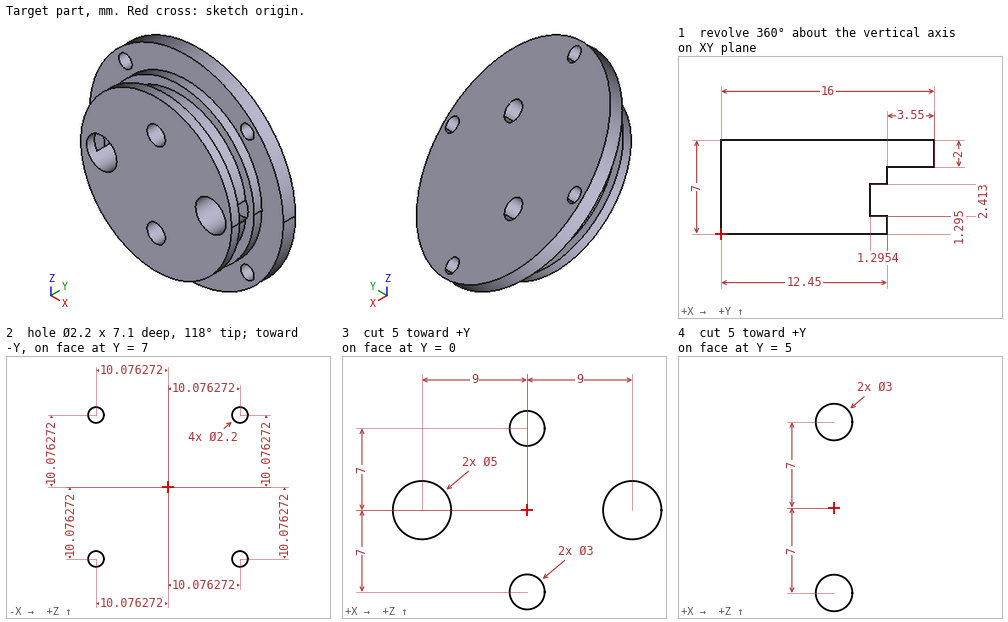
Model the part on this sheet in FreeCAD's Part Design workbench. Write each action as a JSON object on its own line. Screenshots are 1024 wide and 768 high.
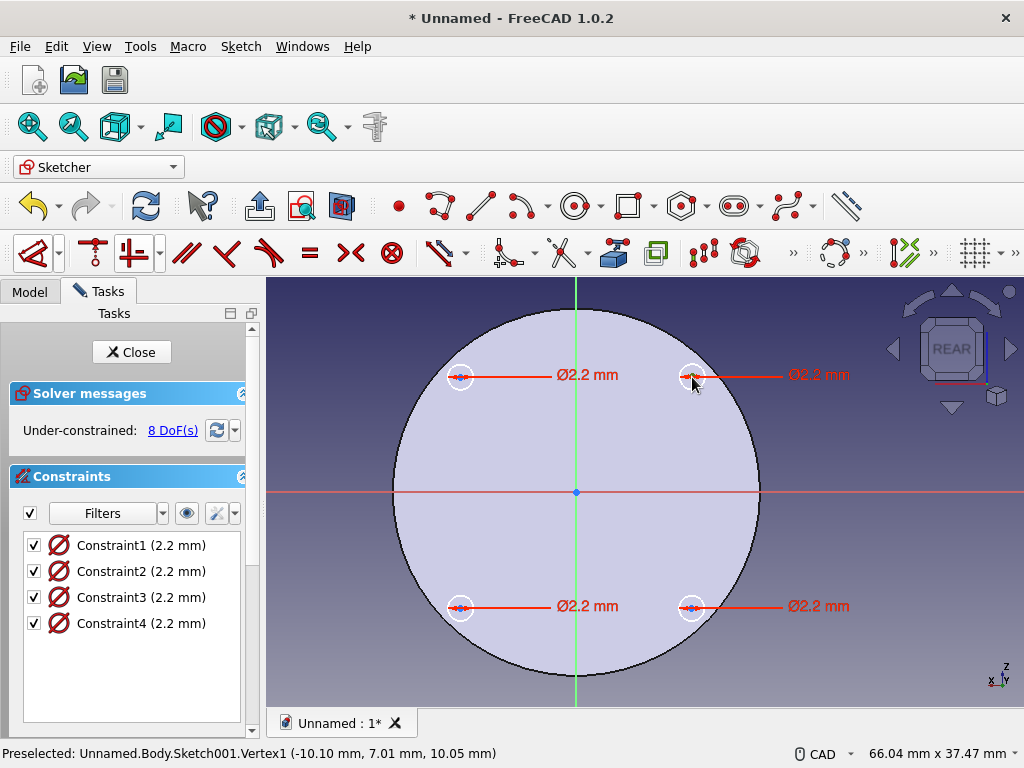
{"action": "key", "text": "l"}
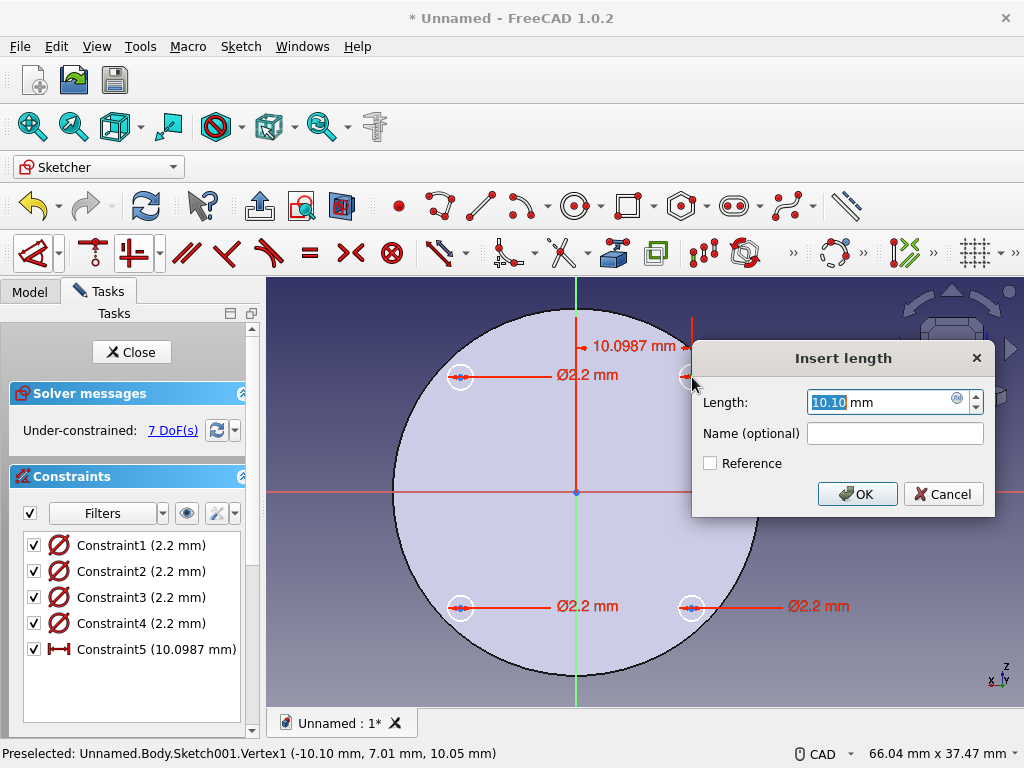
{"action": "type", "text": "10.076272"}
{"action": "key", "text": "Return"}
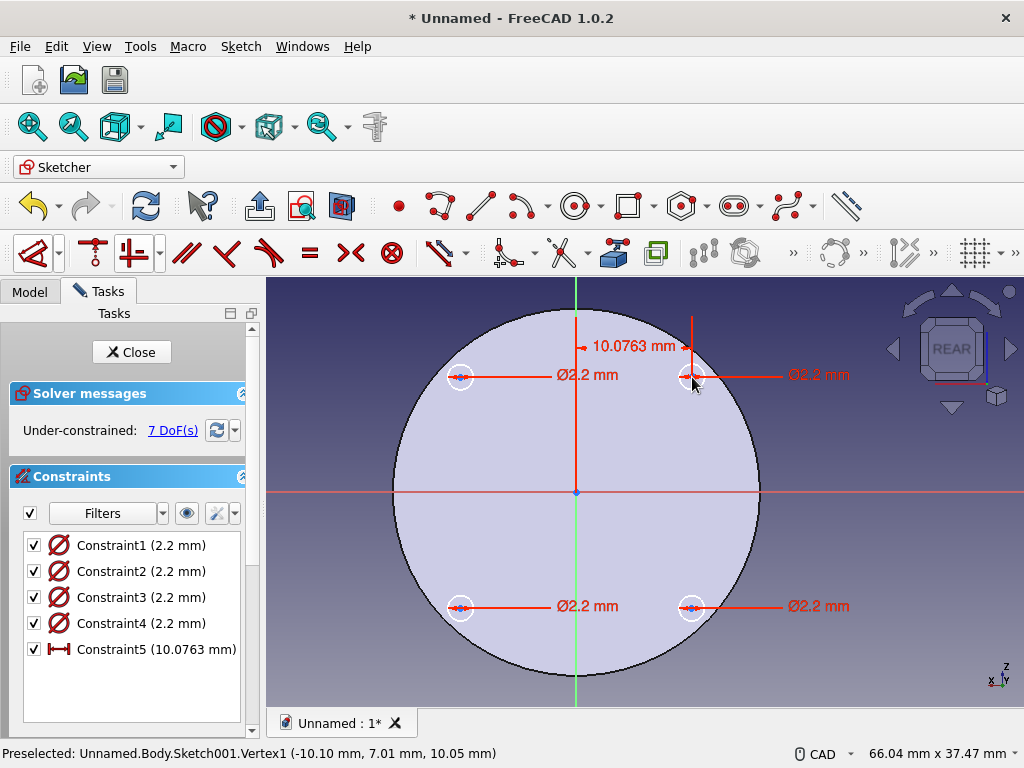
{"action": "left_click", "coordinate": [692, 377]}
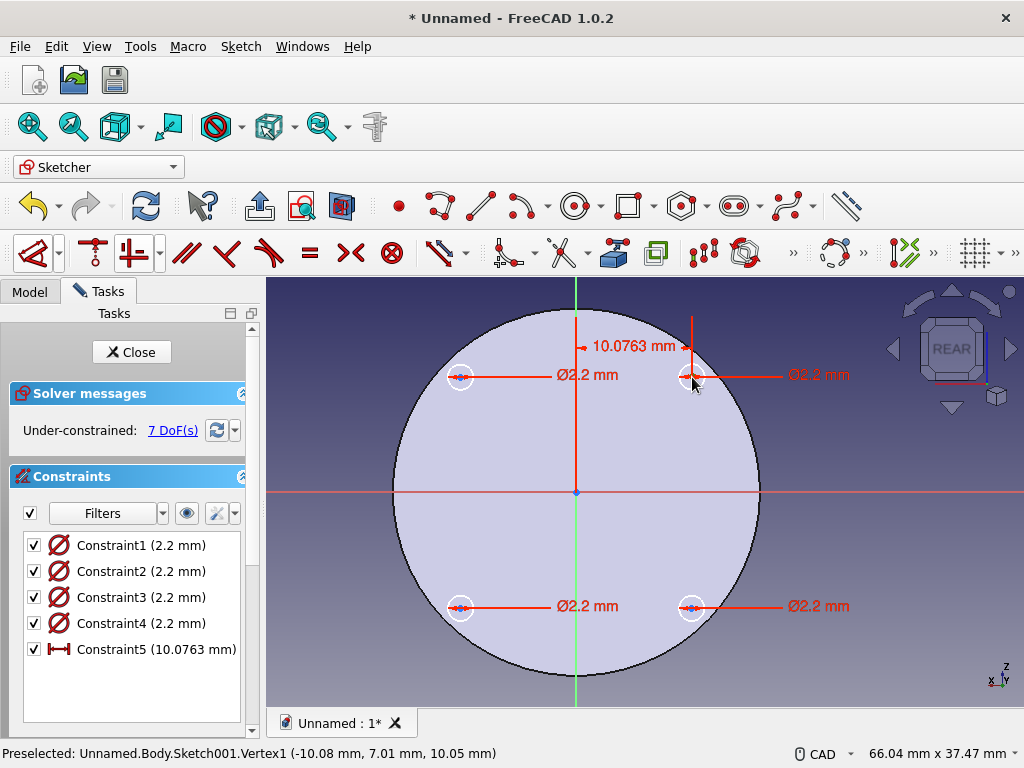
{"action": "left_click", "coordinate": [58, 254]}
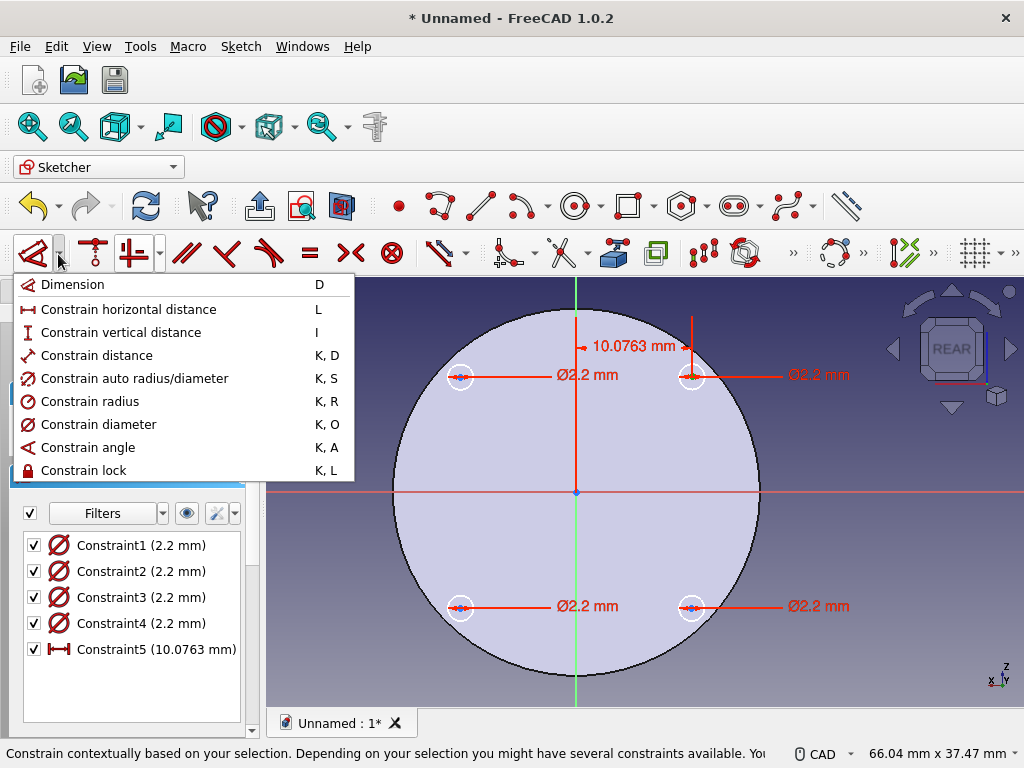
{"action": "left_click", "coordinate": [184, 332]}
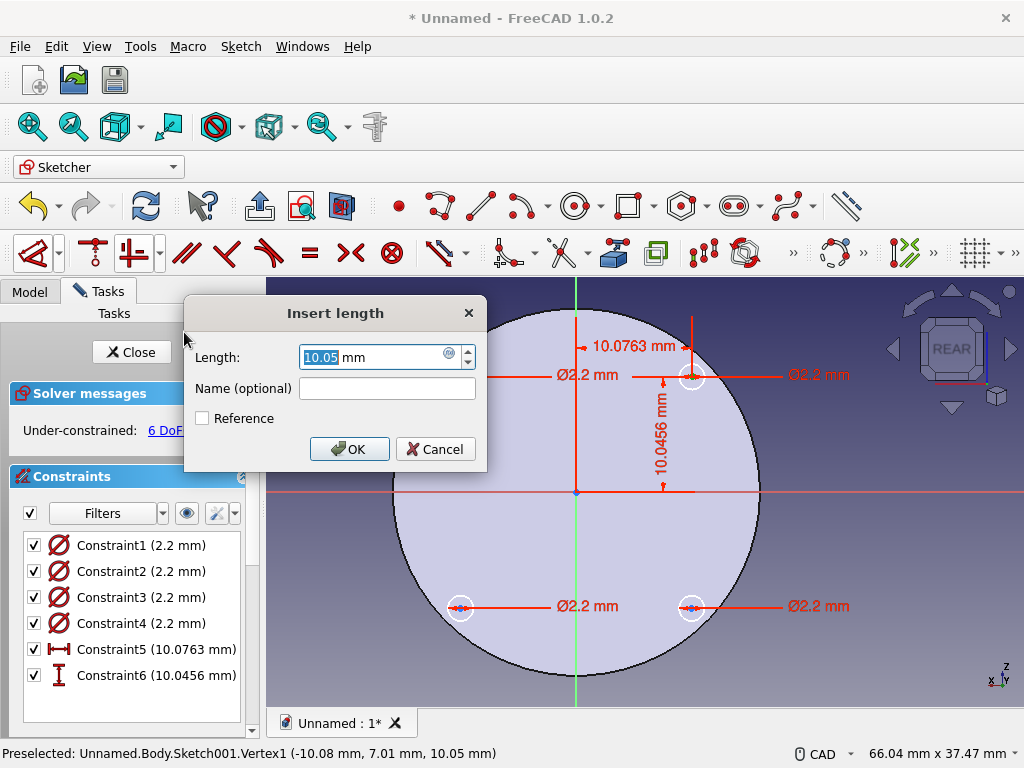
{"action": "type", "text": "10.076272"}
{"action": "key", "text": "Return"}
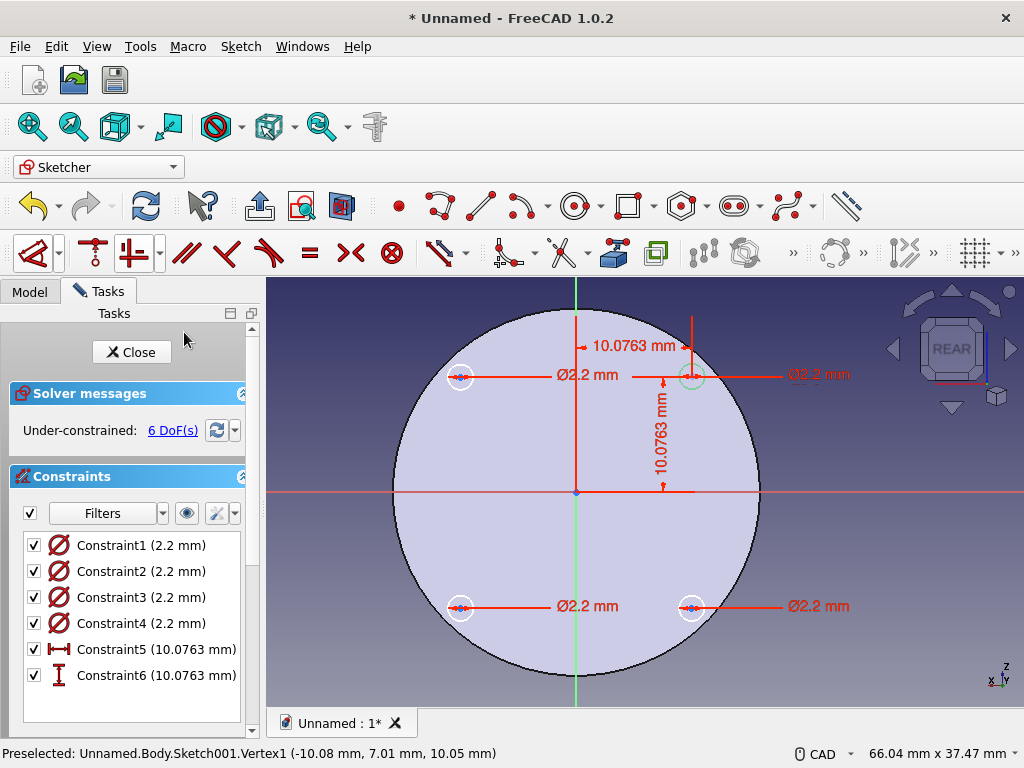
{"action": "left_click", "coordinate": [692, 608]}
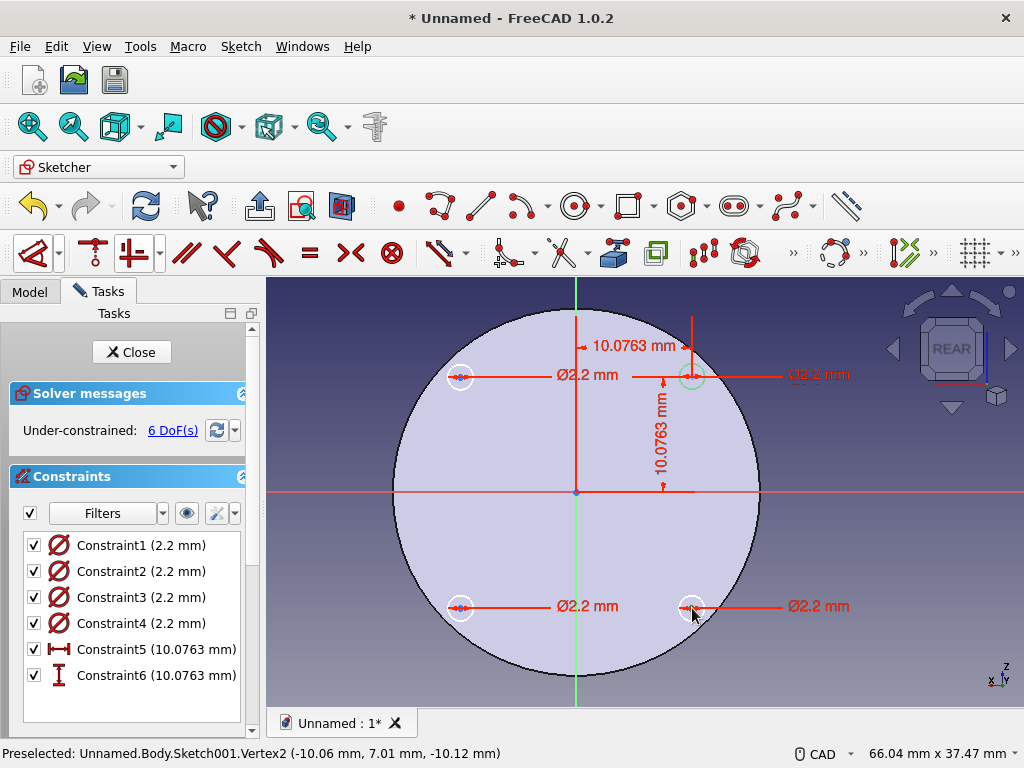
{"action": "left_click", "coordinate": [58, 254]}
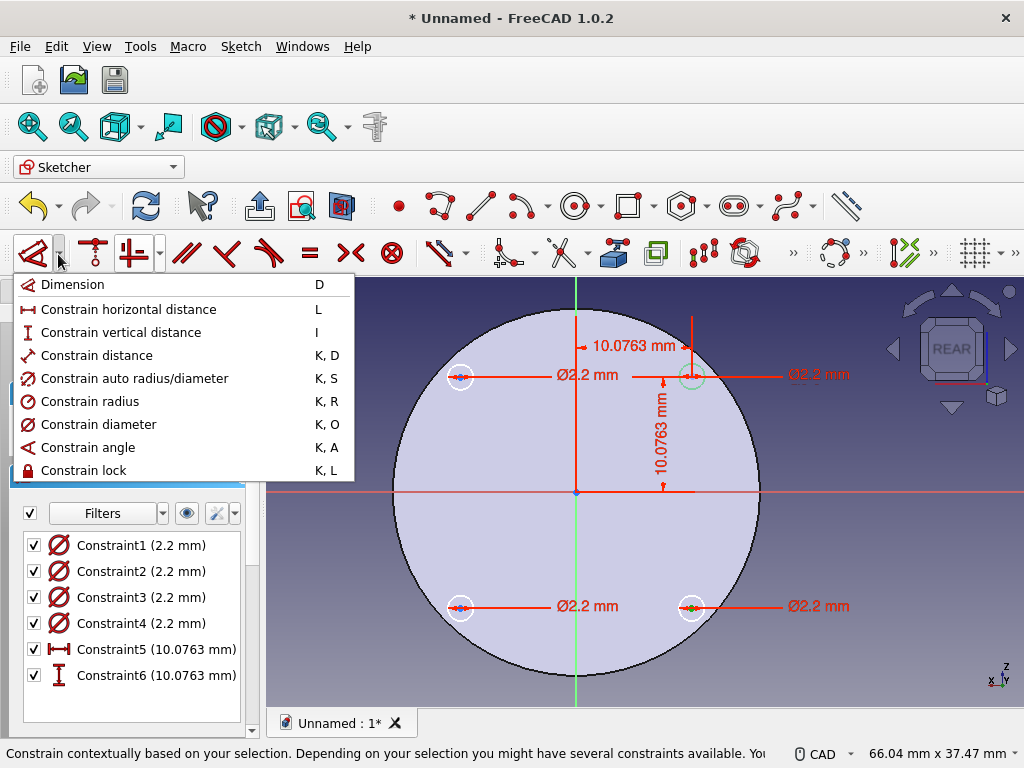
{"action": "left_click", "coordinate": [184, 310]}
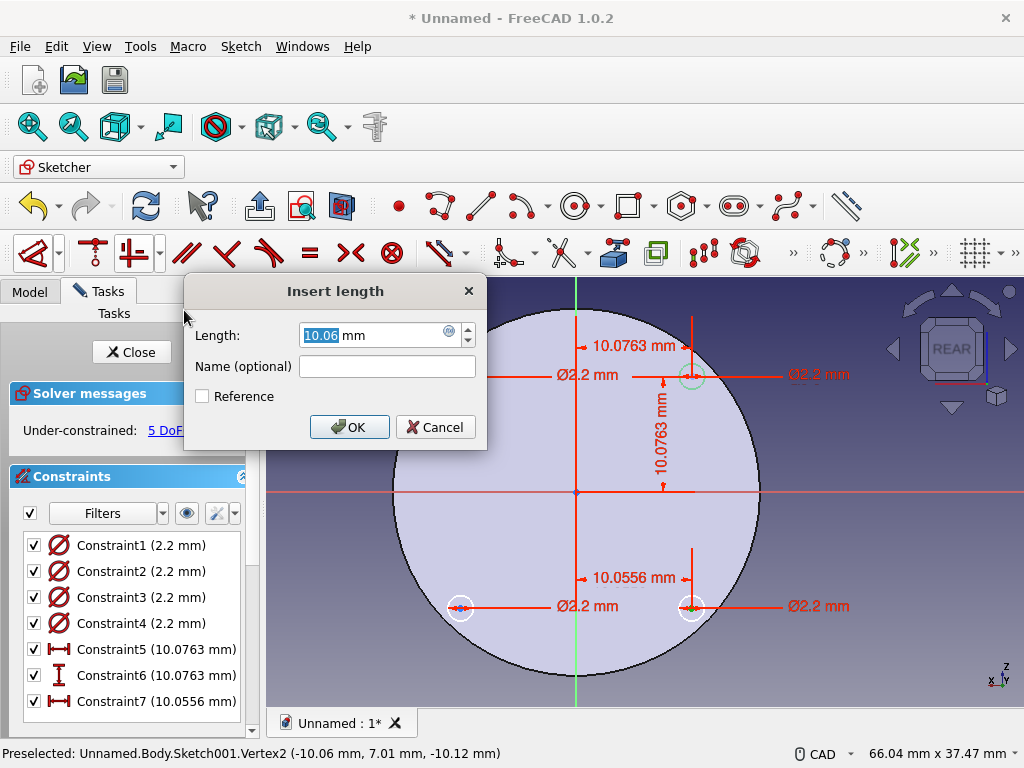
{"action": "type", "text": "10.076272"}
{"action": "key", "text": "Return"}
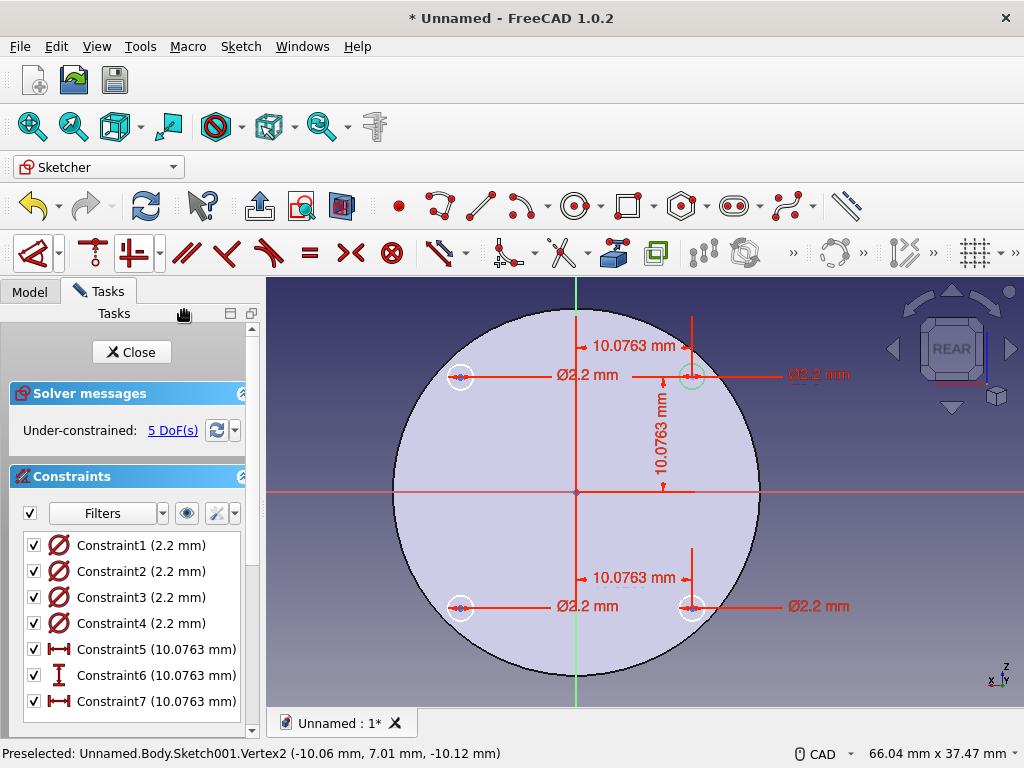
{"action": "left_click", "coordinate": [692, 608]}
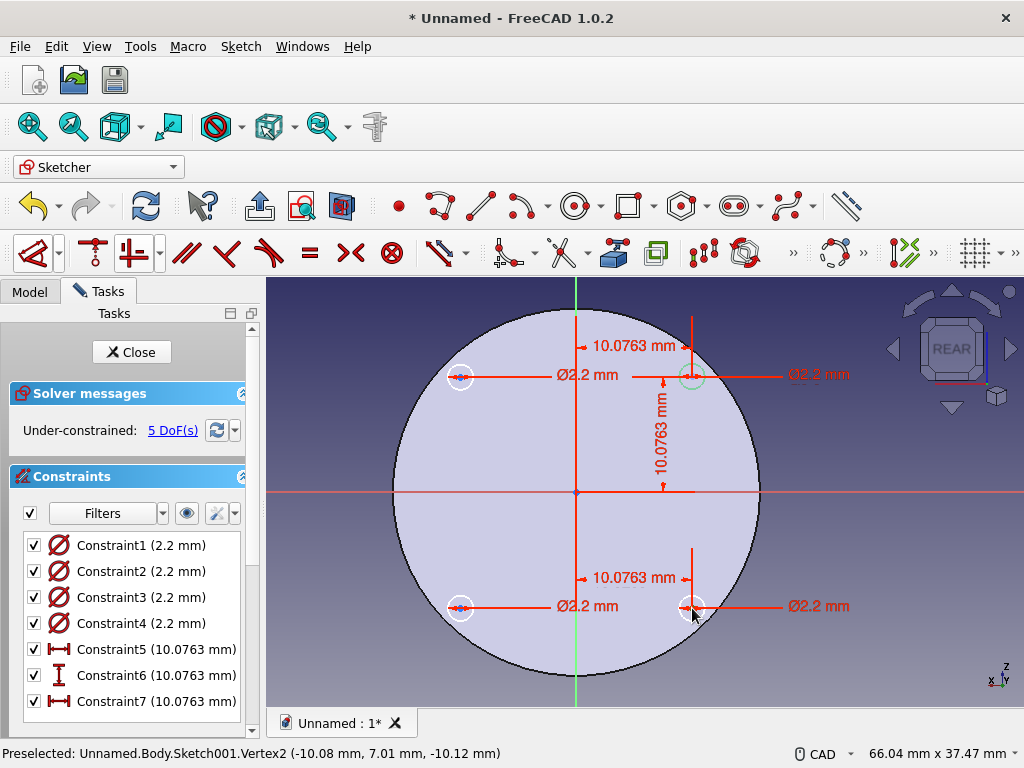
{"action": "left_click", "coordinate": [58, 254]}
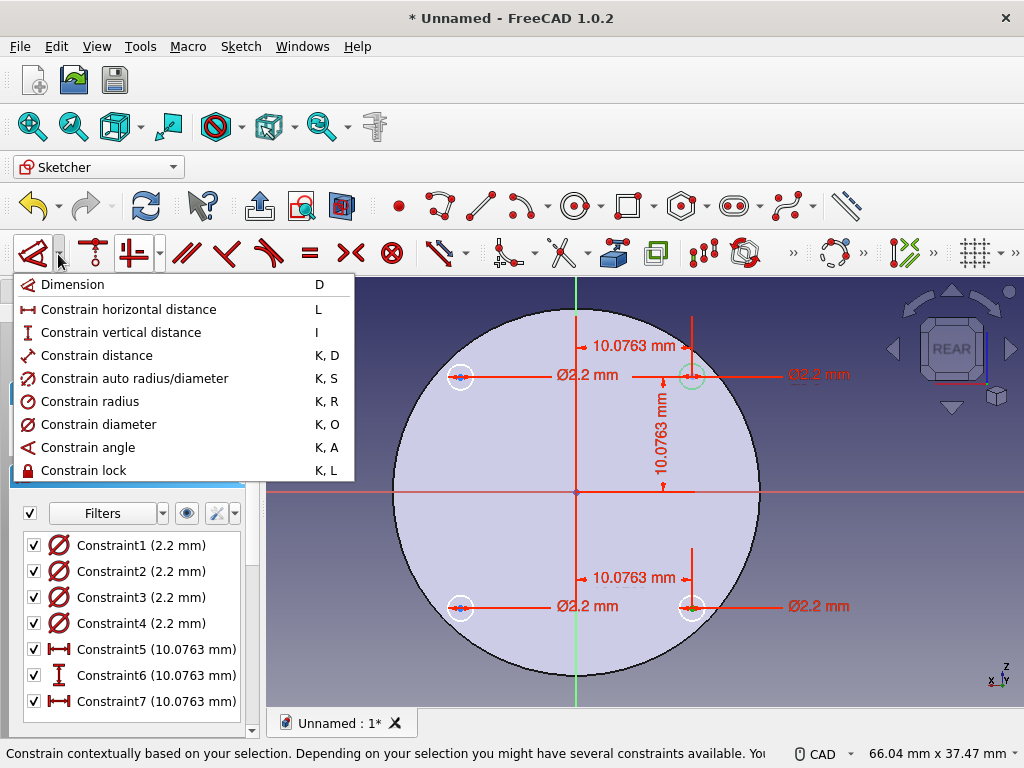
{"action": "left_click", "coordinate": [184, 332]}